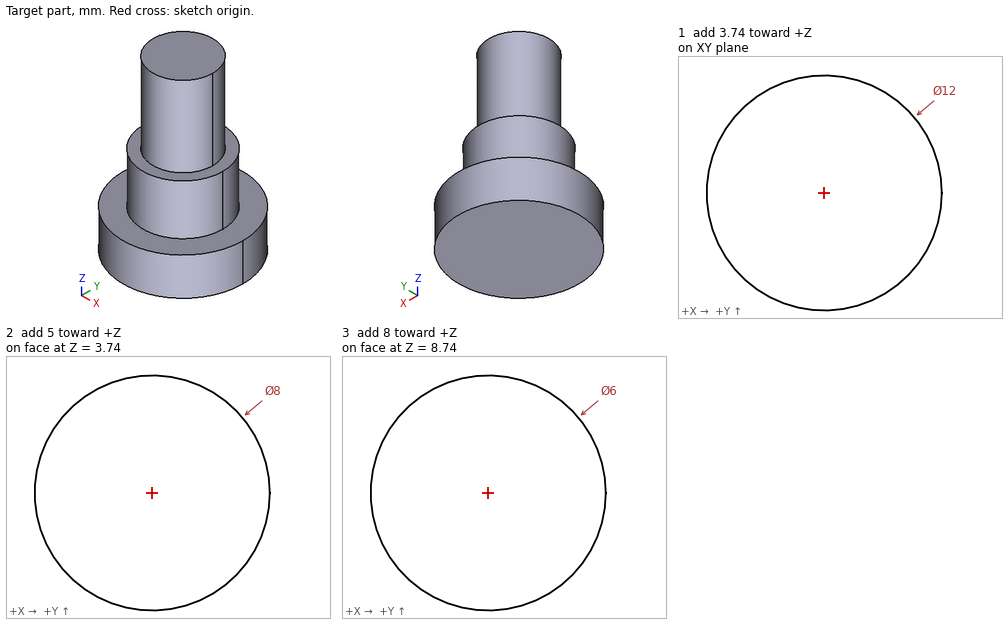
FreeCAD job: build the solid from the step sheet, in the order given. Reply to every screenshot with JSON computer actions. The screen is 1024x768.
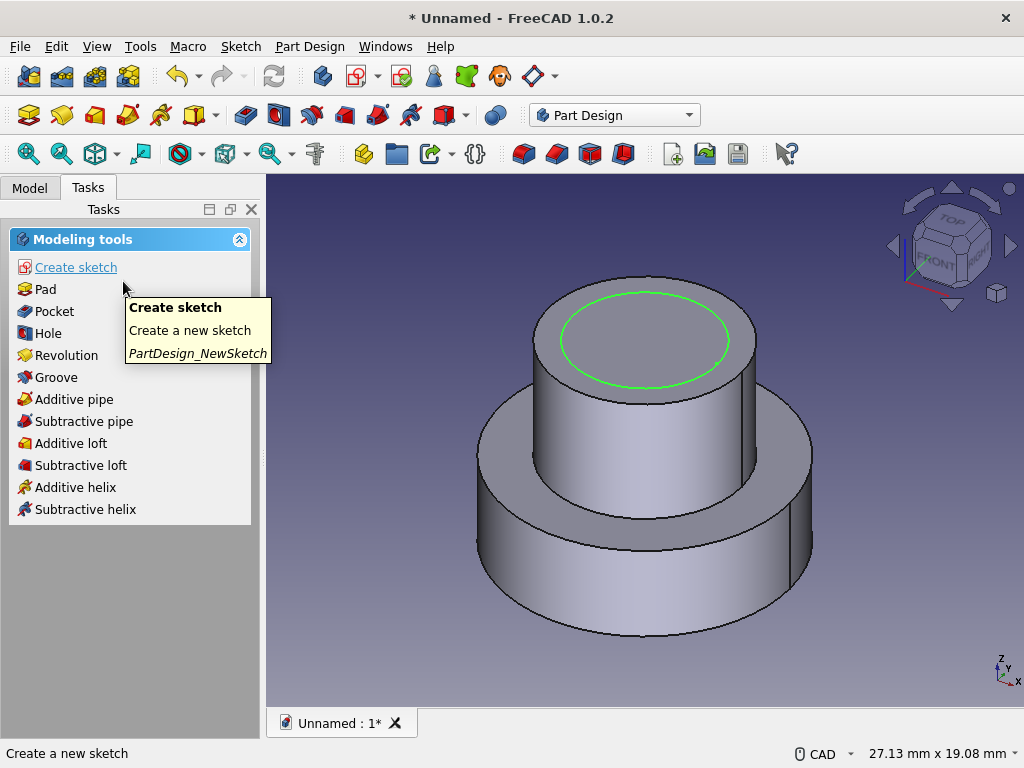
{"action": "left_click", "coordinate": [29, 116]}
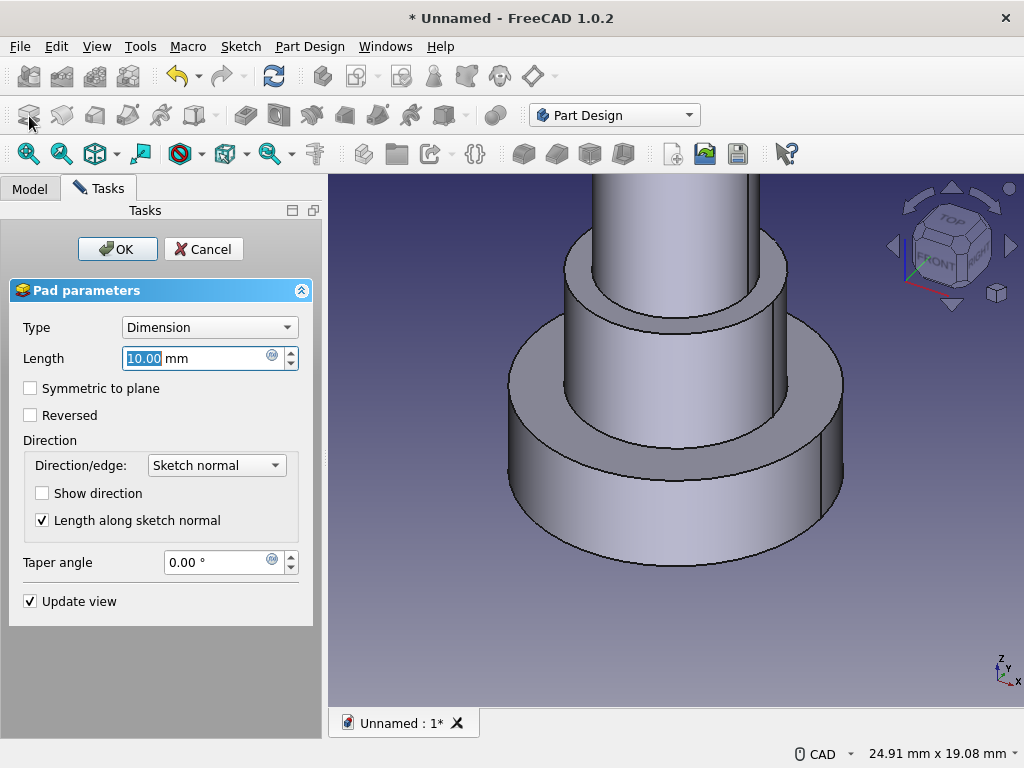
{"action": "type", "text": "8"}
{"action": "key", "text": "Tab"}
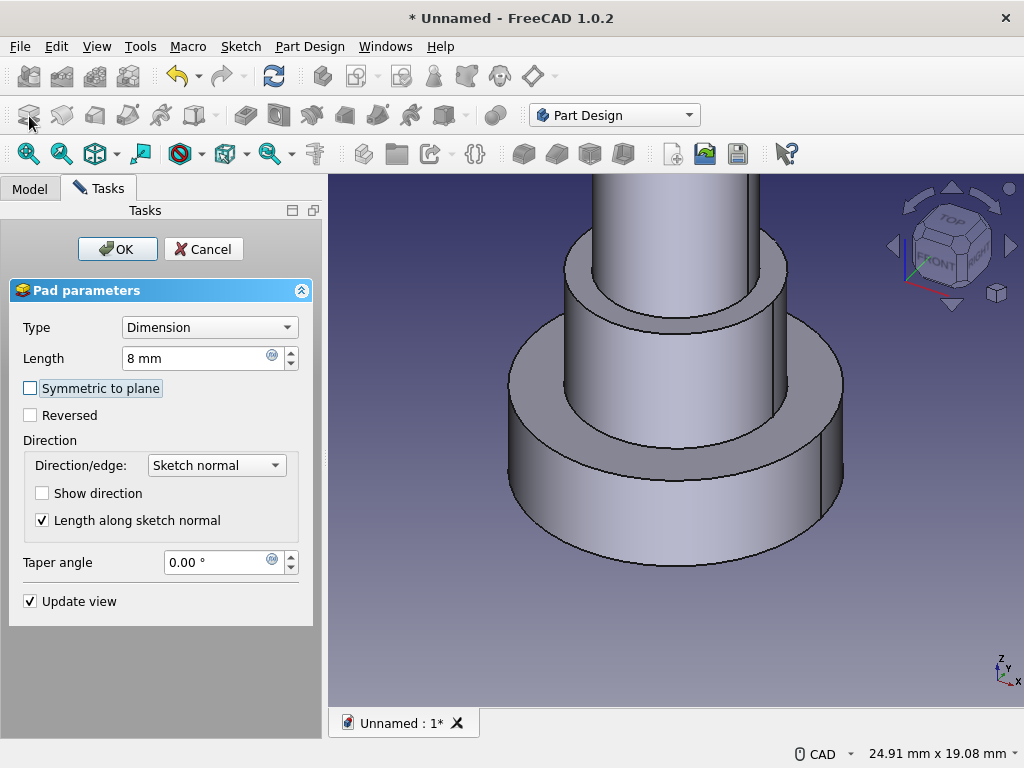
{"action": "left_click", "coordinate": [118, 249]}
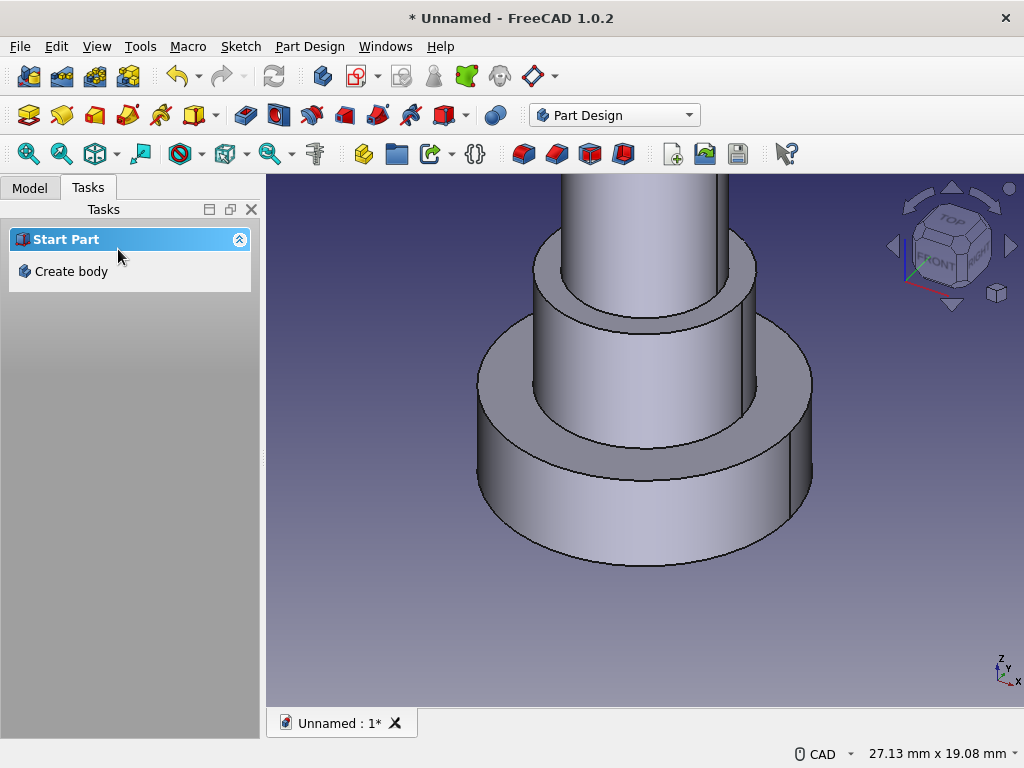
{"action": "key", "text": "0"}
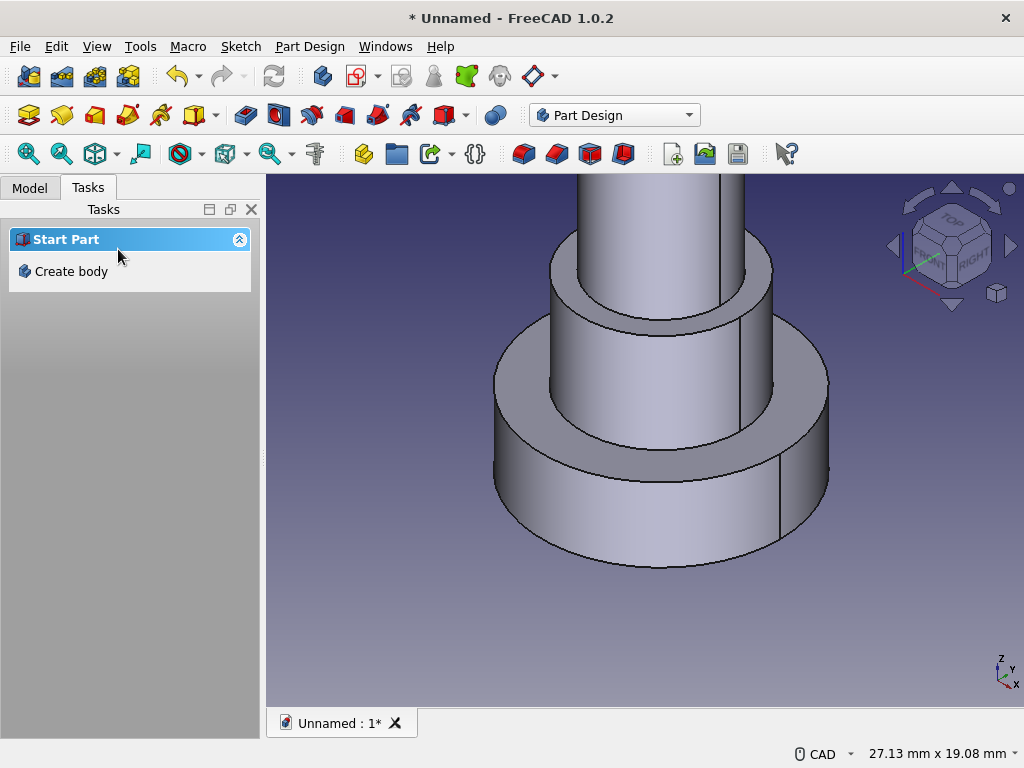
{"action": "left_click", "coordinate": [29, 154]}